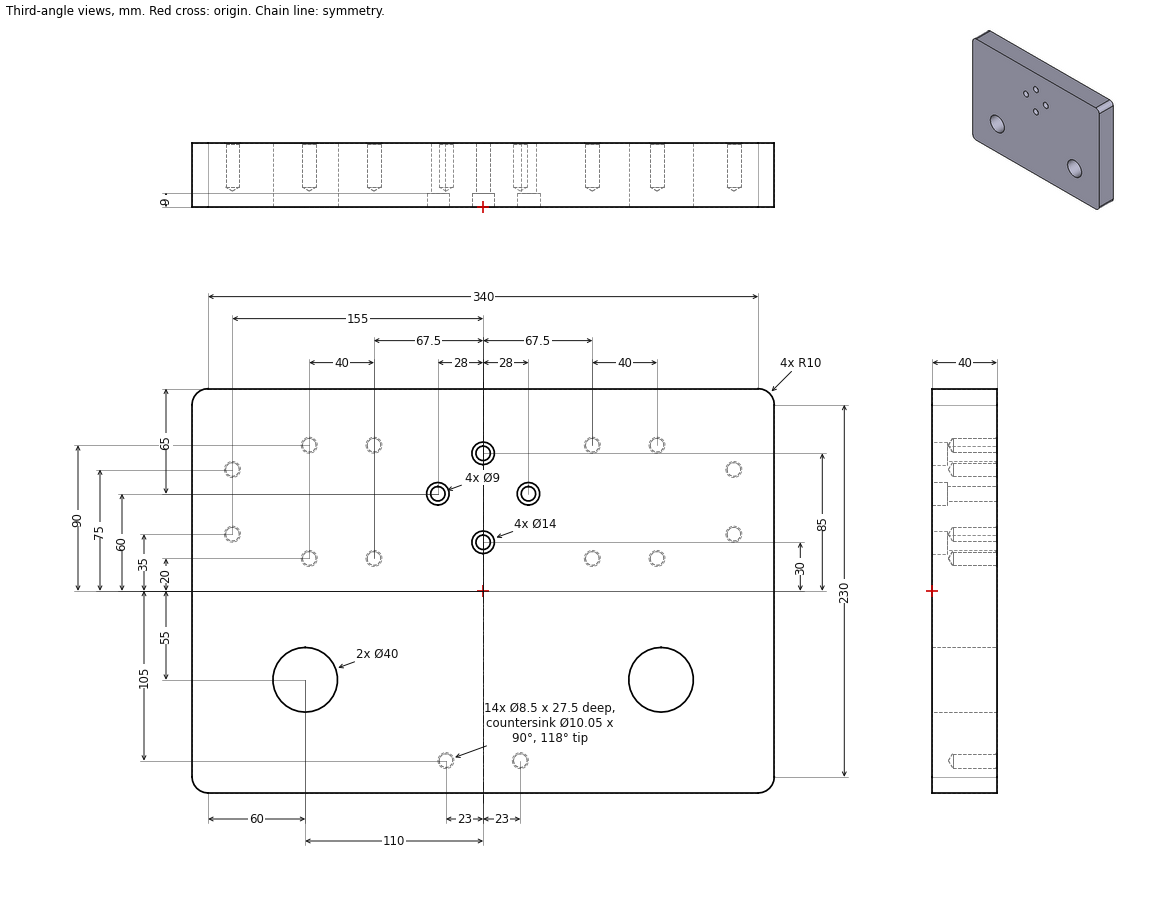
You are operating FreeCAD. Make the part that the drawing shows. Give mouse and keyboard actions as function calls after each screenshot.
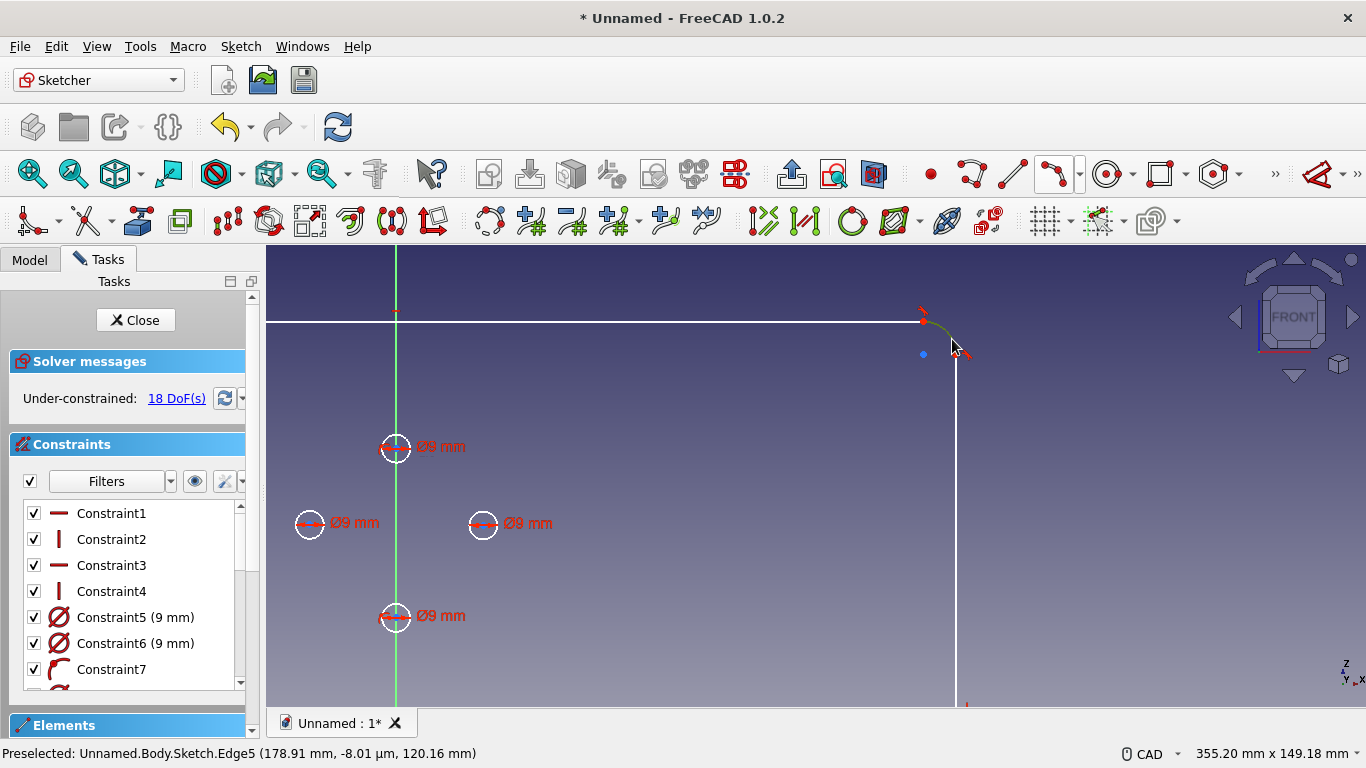
scroll(952, 341, down, 5)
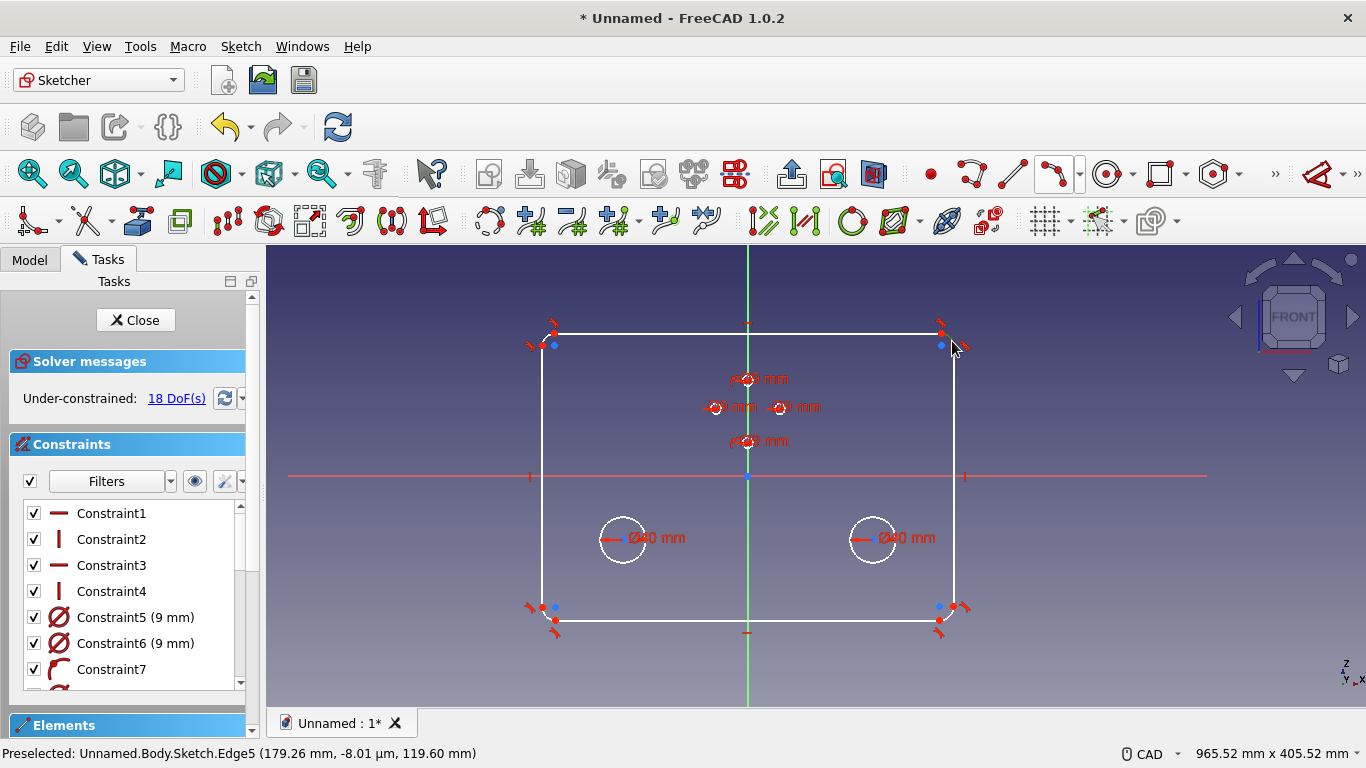
scroll(946, 619, up, 4)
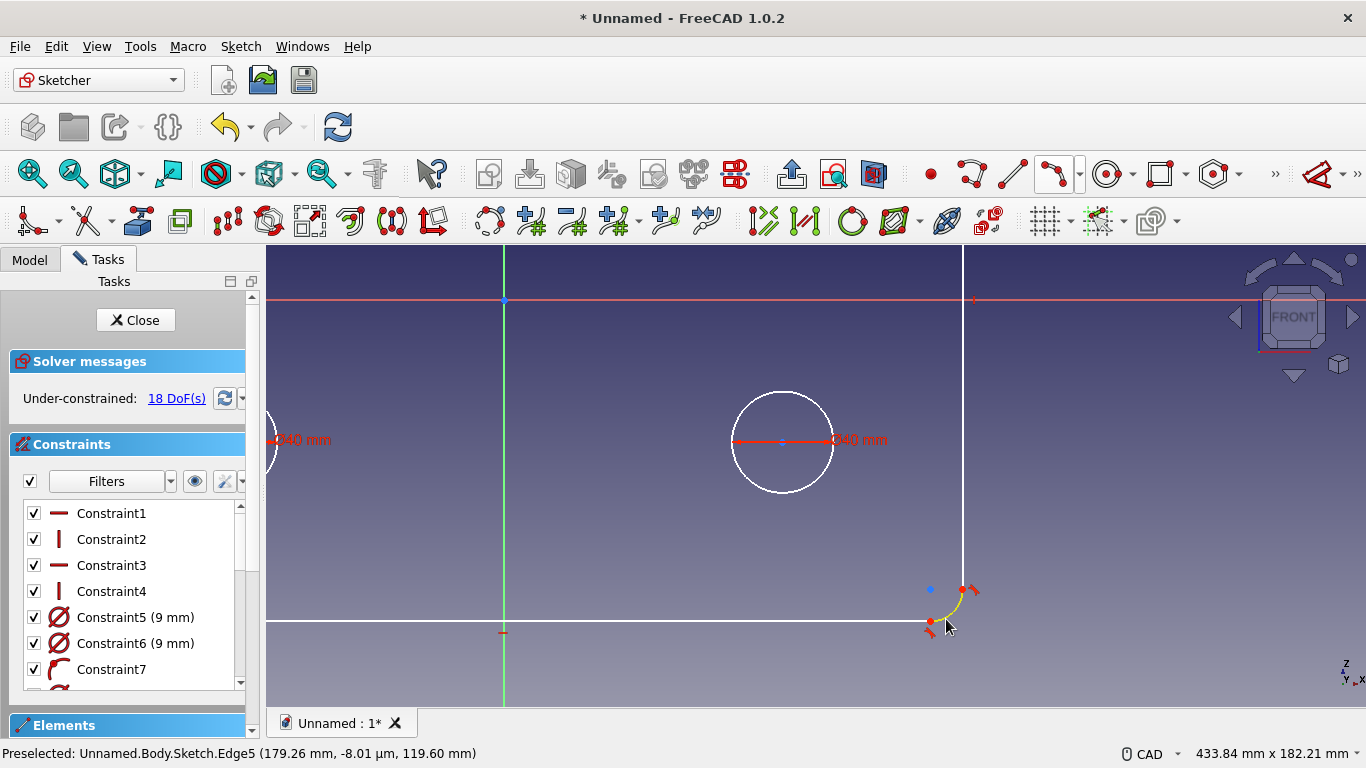
click(945, 618)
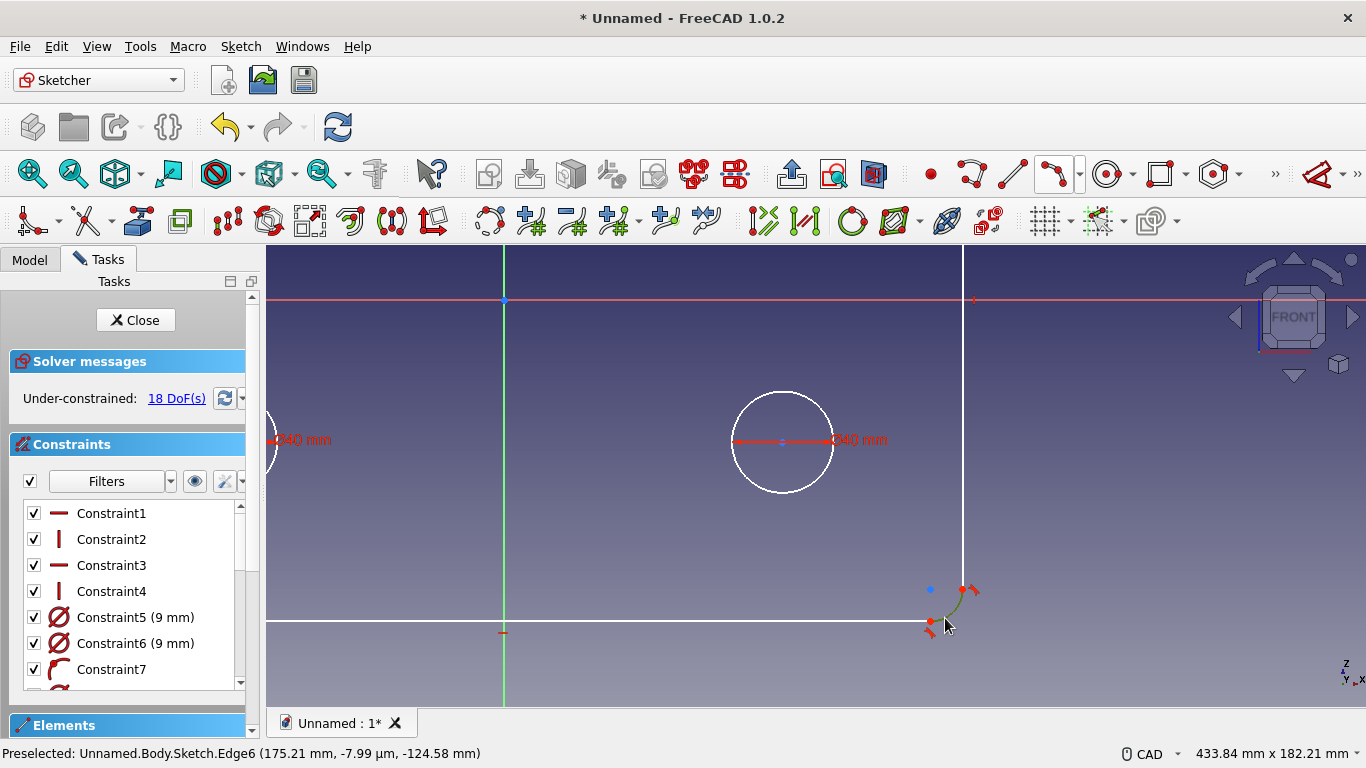
scroll(946, 620, down, 4)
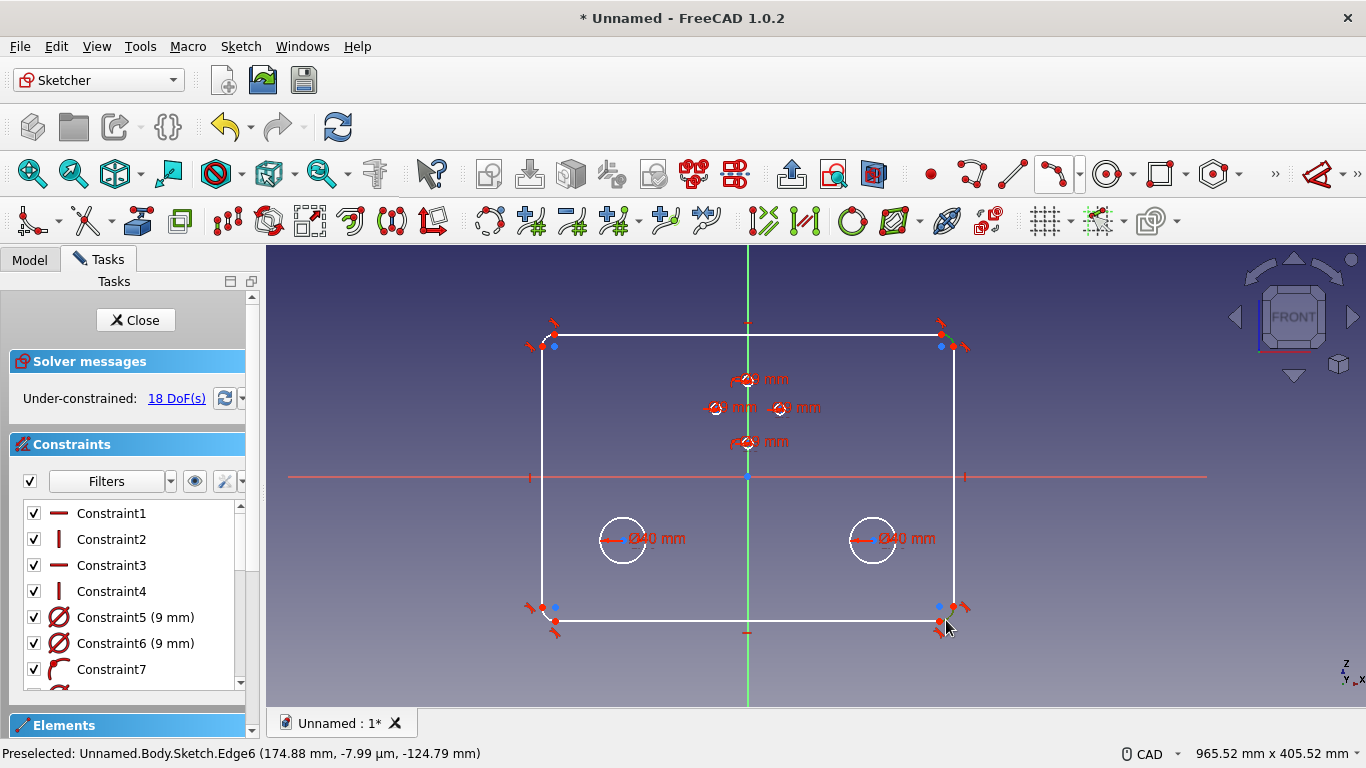
scroll(544, 614, up, 4)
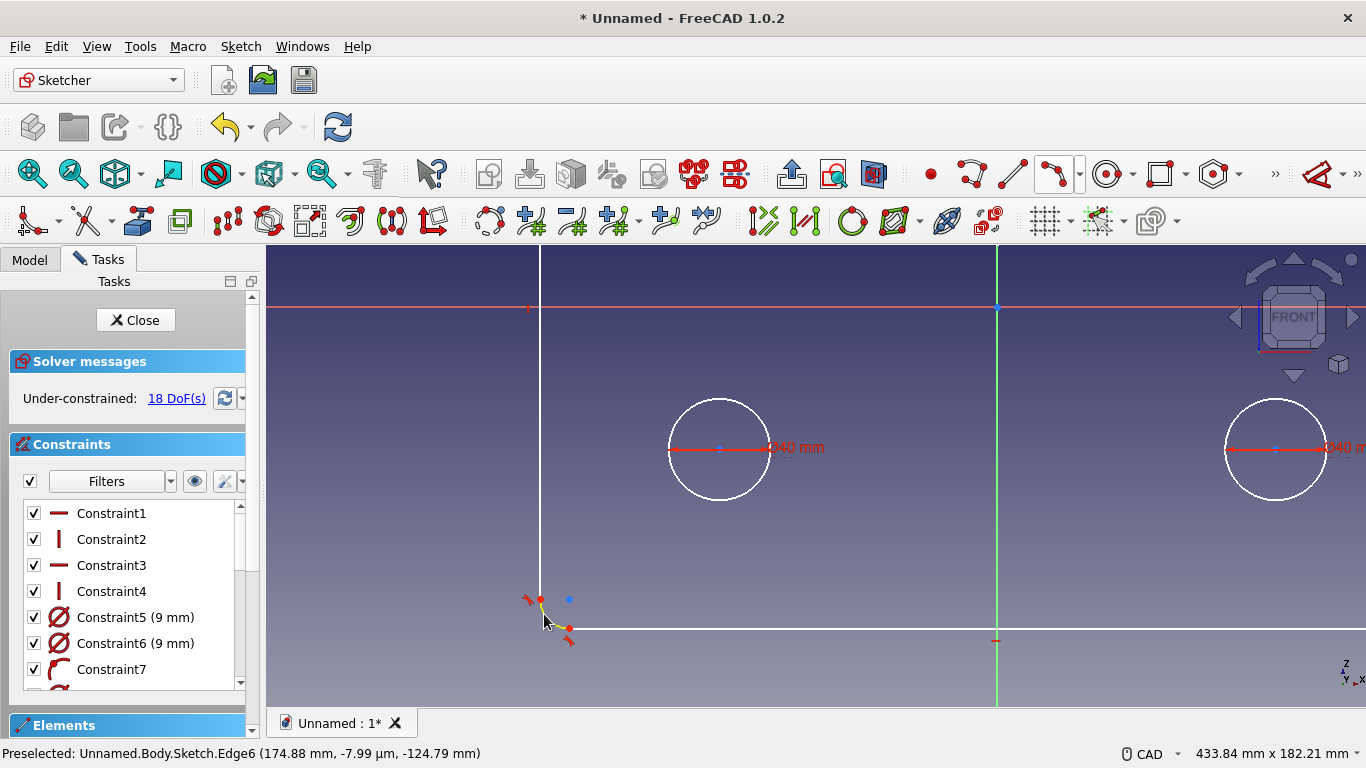
click(543, 613)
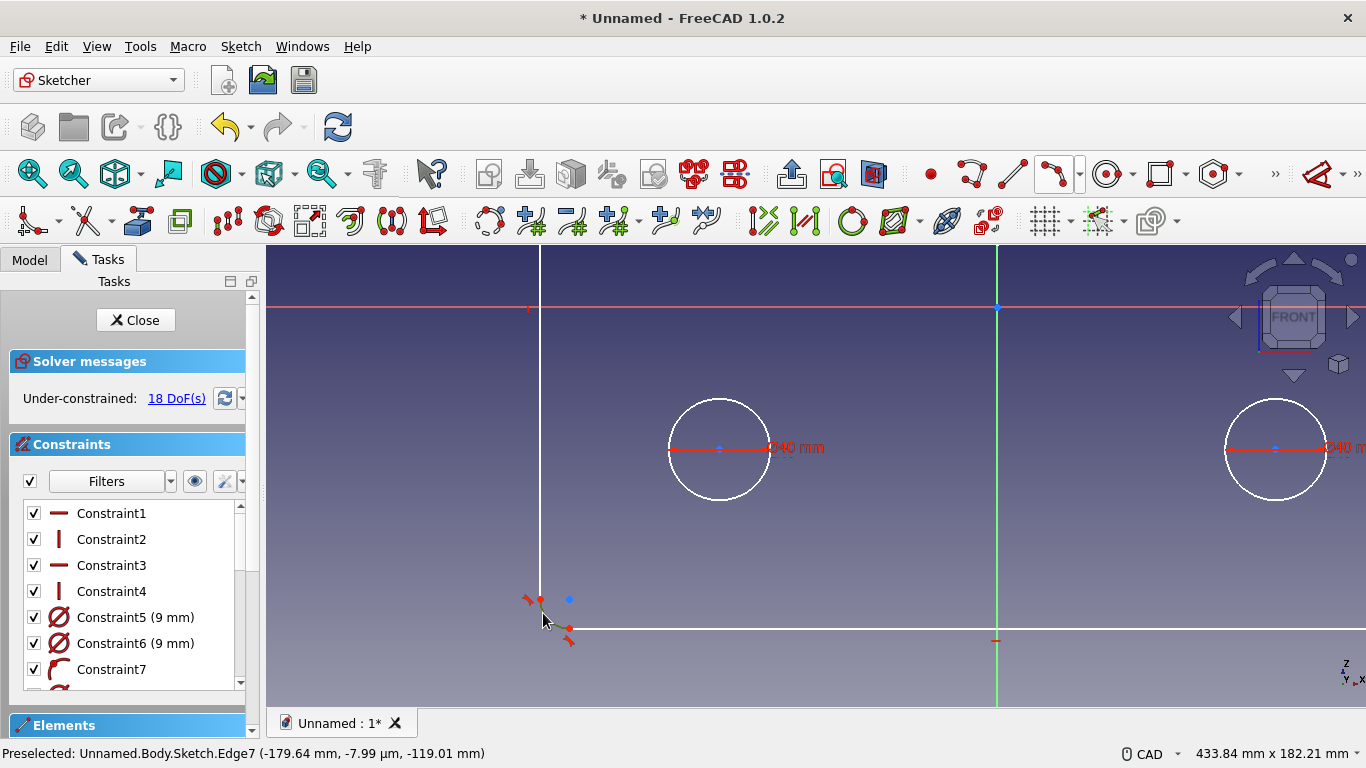
scroll(544, 614, down, 4)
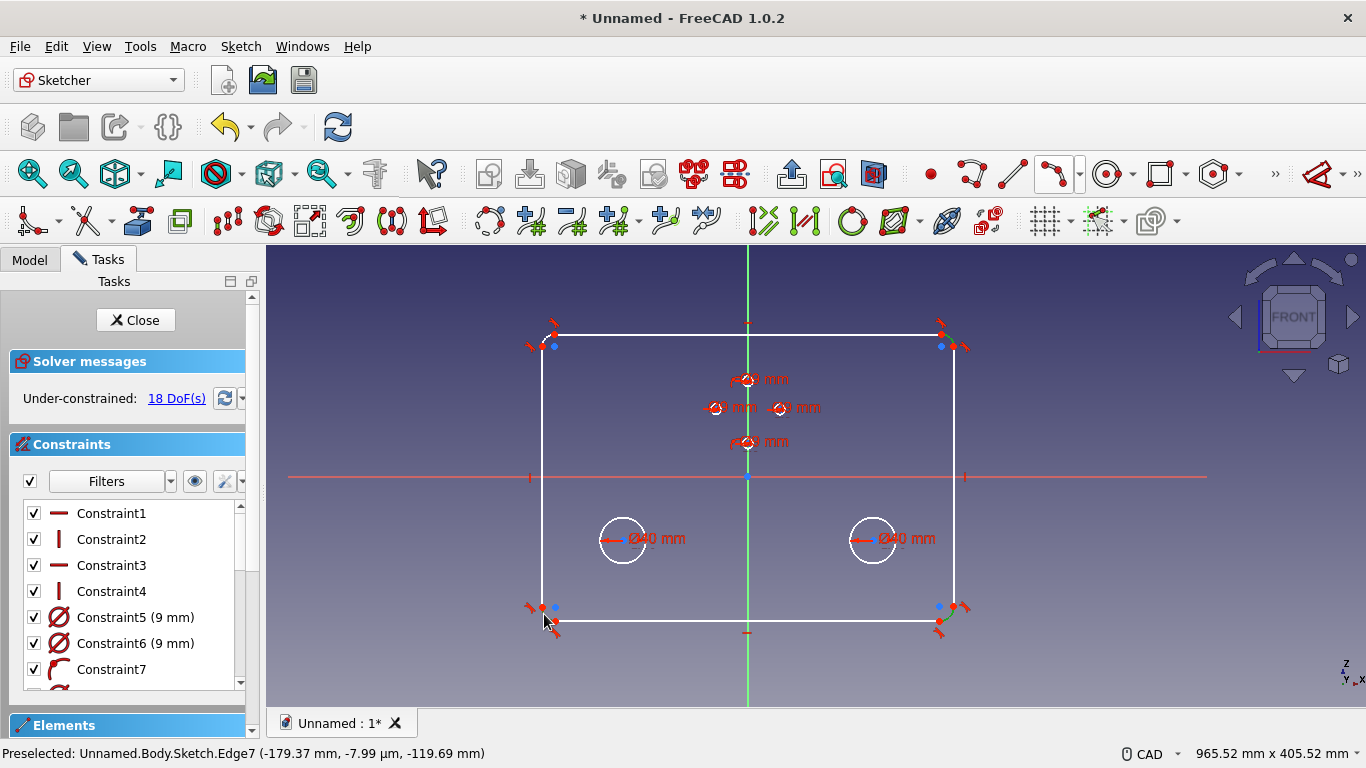
scroll(549, 336, up, 5)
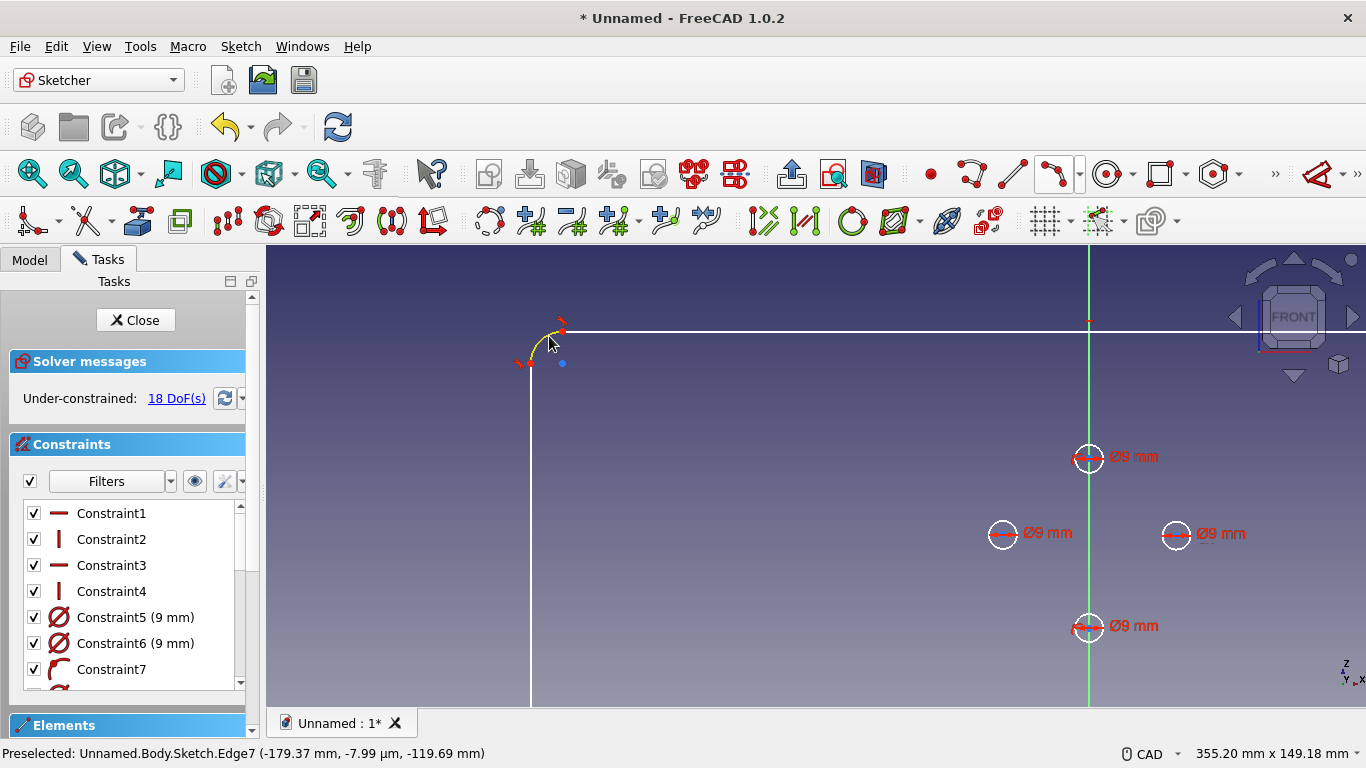
click(548, 335)